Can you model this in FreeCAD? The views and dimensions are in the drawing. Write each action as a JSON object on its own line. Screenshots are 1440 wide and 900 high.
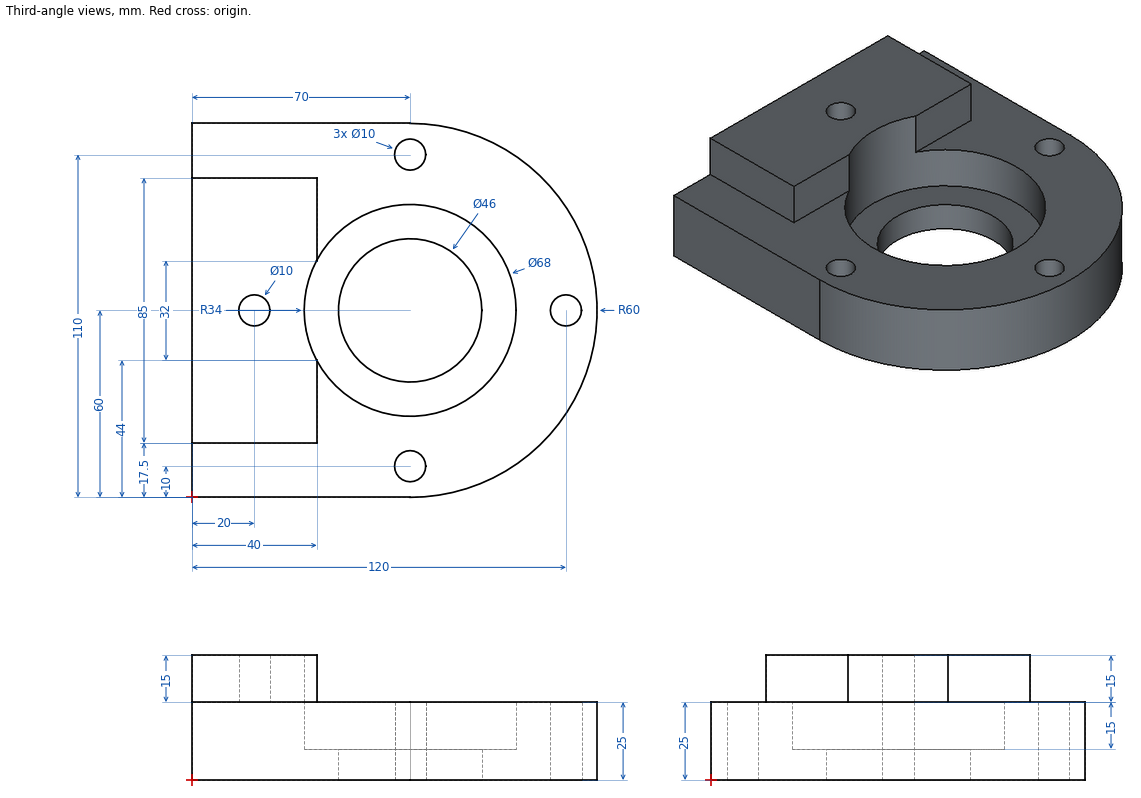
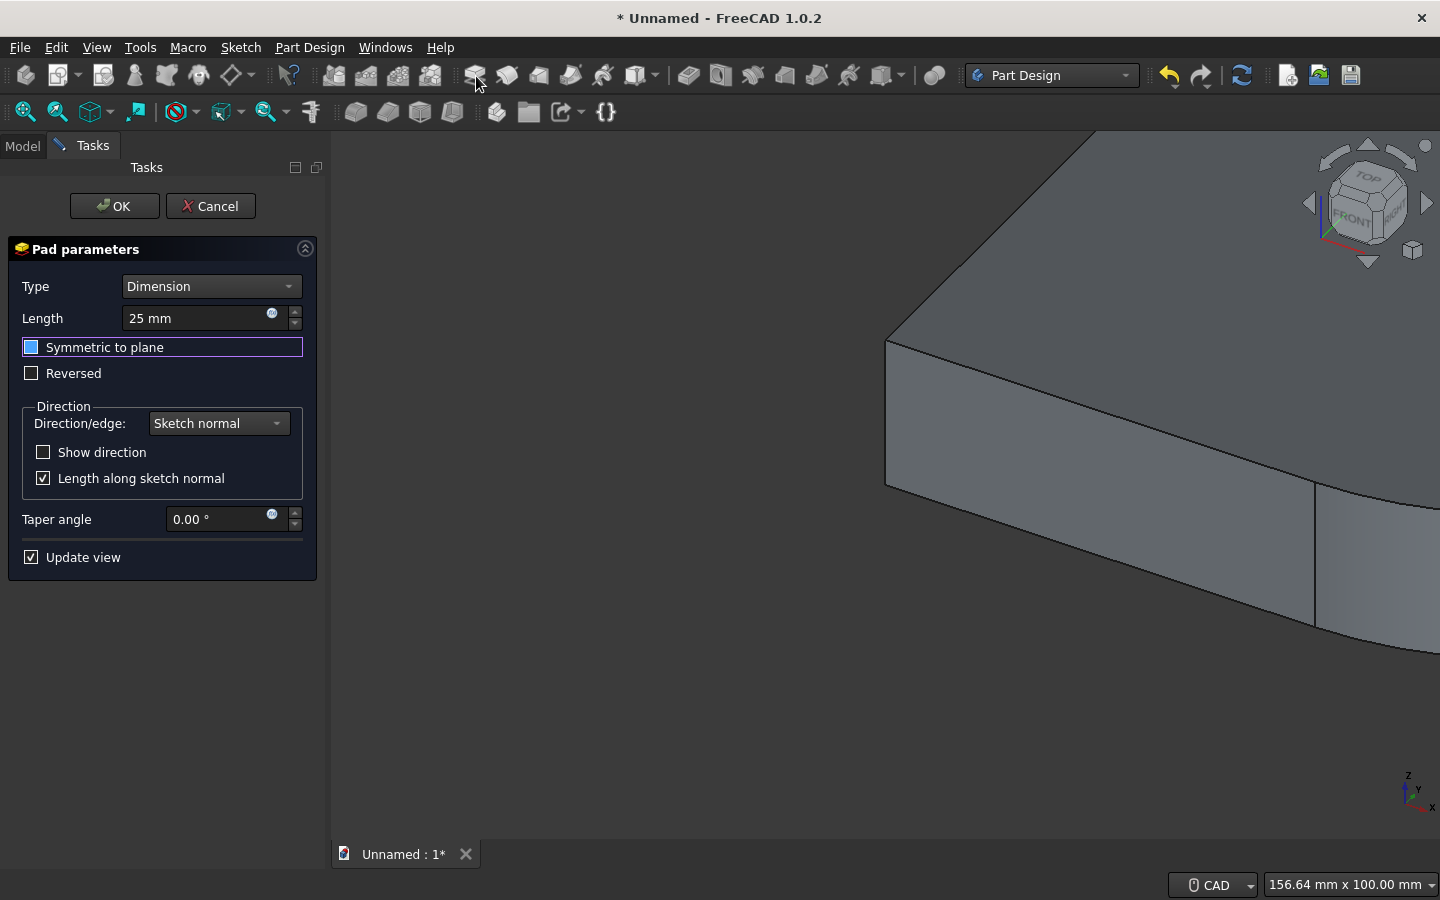
{"action": "left_click", "coordinate": [115, 206]}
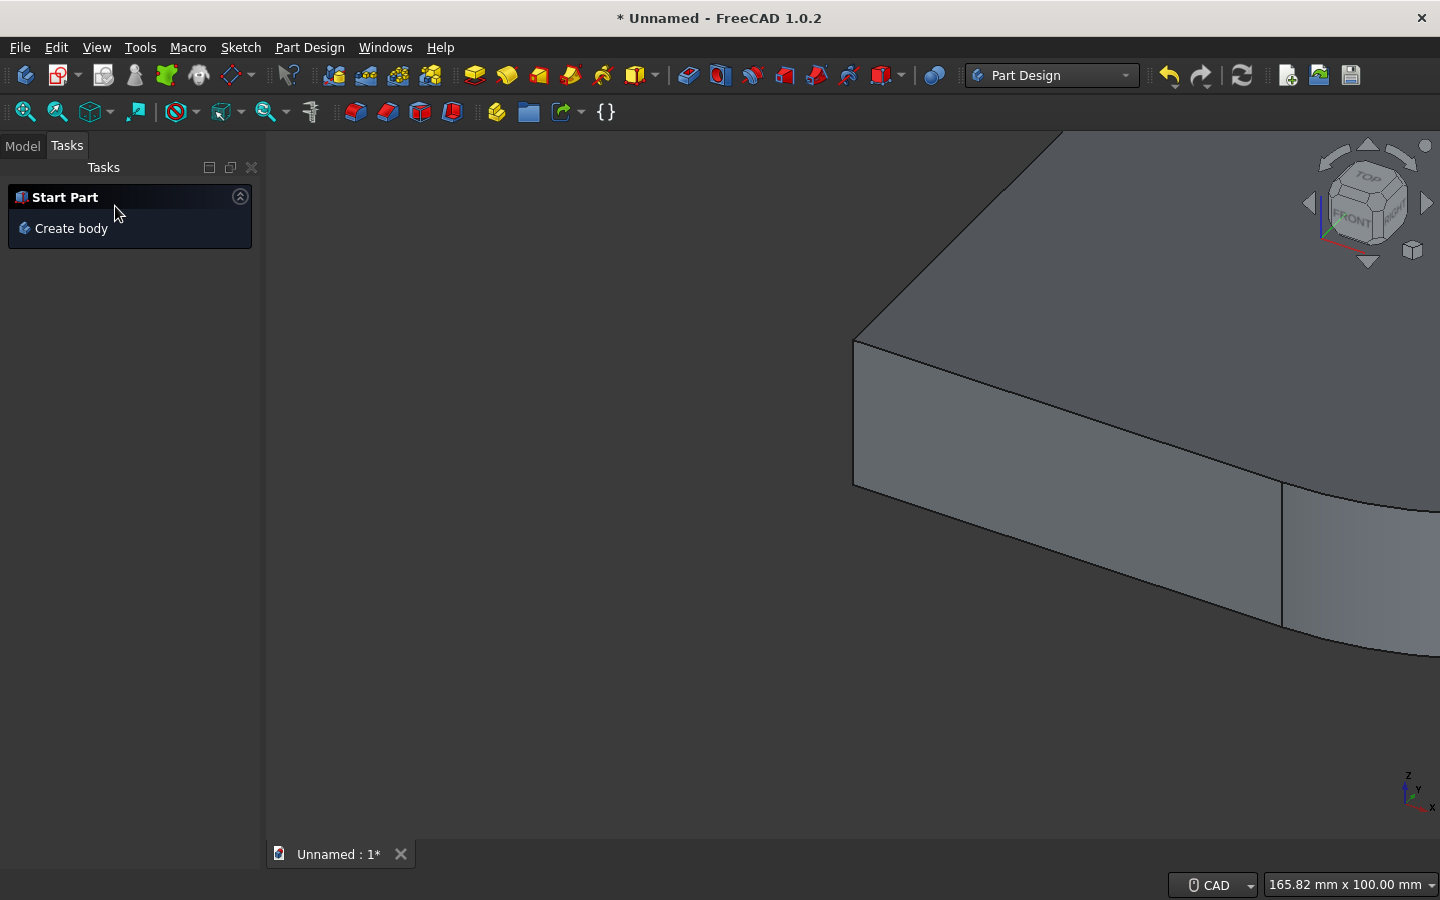
{"action": "left_click", "coordinate": [26, 112]}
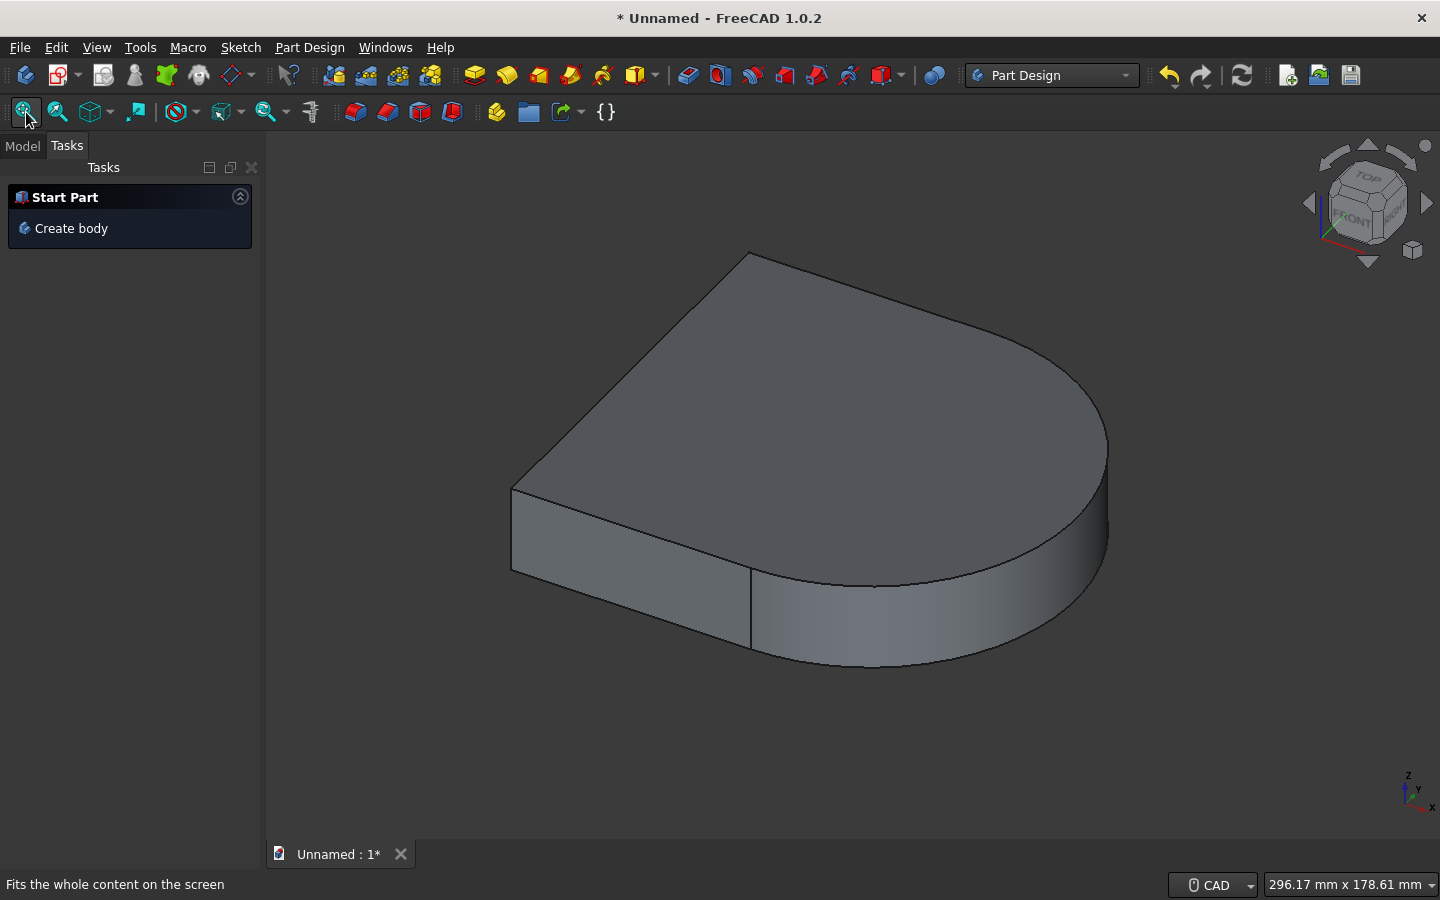
{"action": "left_click", "coordinate": [853, 443]}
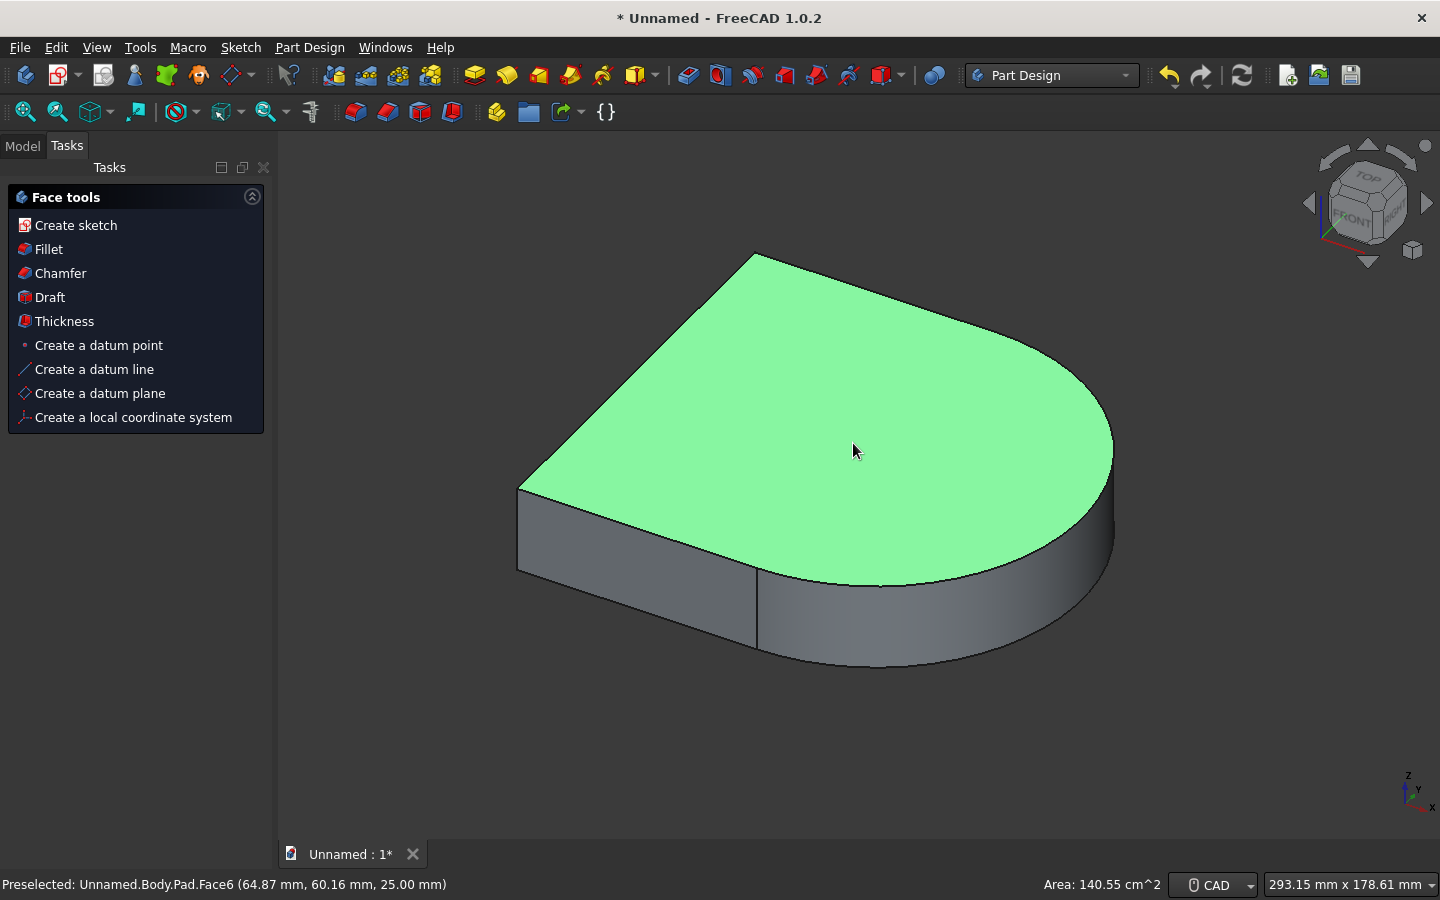
{"action": "left_click", "coordinate": [58, 76]}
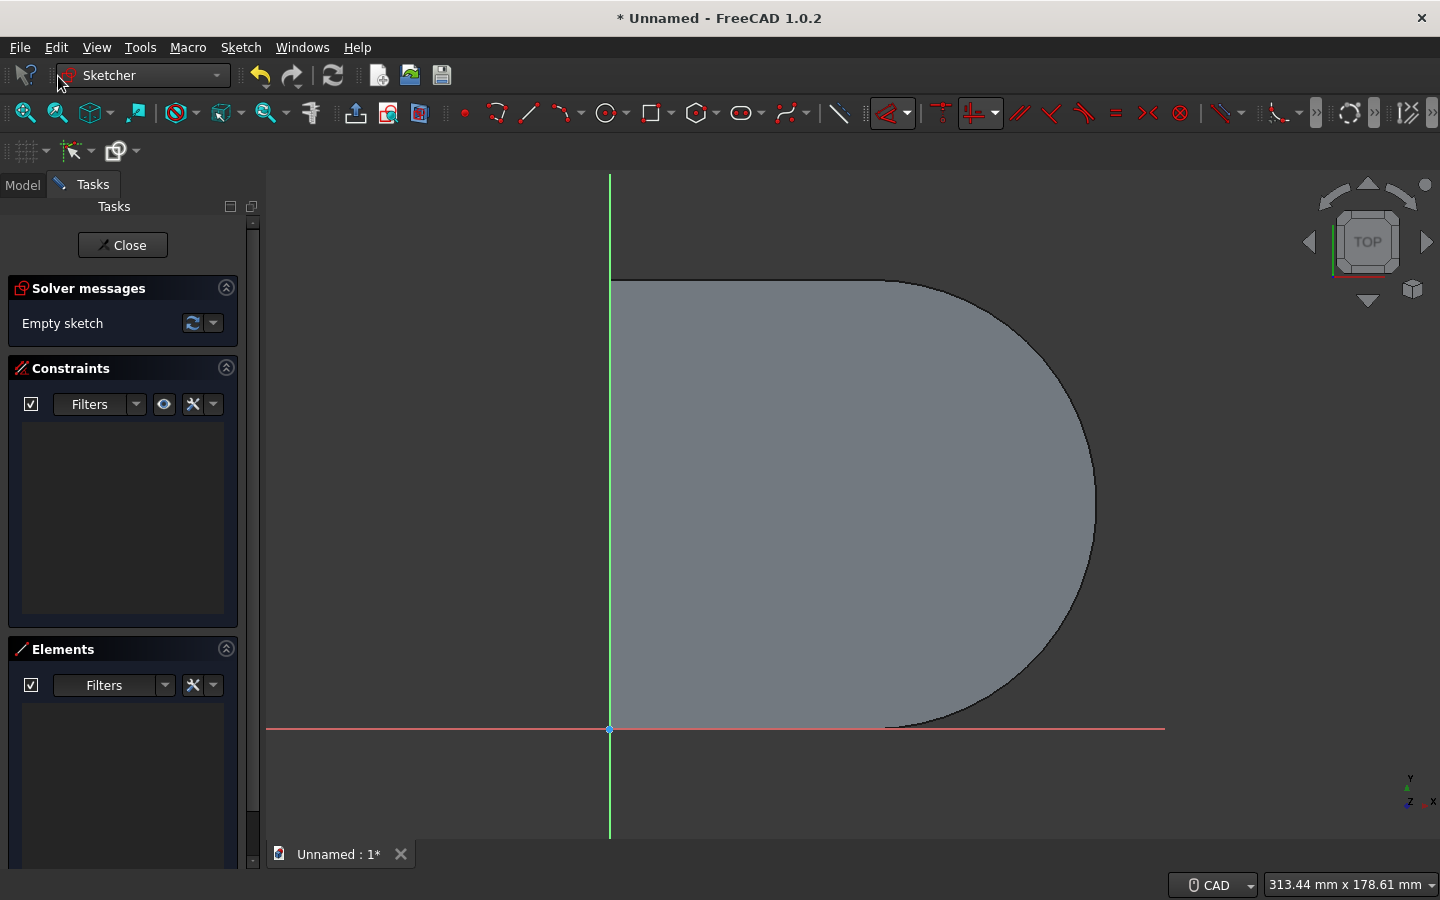
{"action": "key", "text": "g r"}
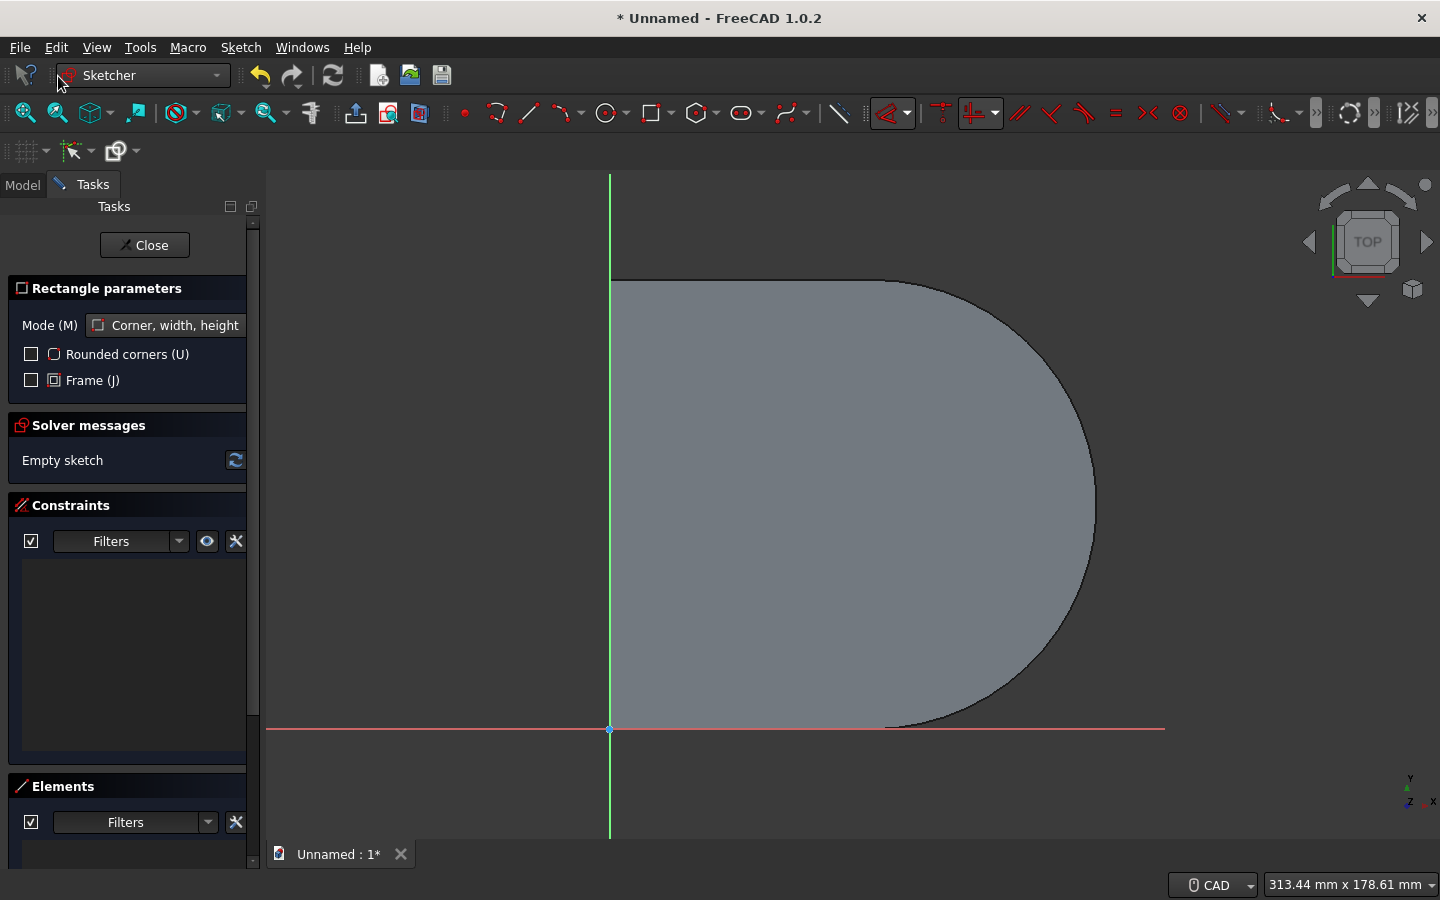
{"action": "left_click", "coordinate": [610, 345]}
{"action": "left_click", "coordinate": [760, 664]}
{"action": "key", "text": "Escape"}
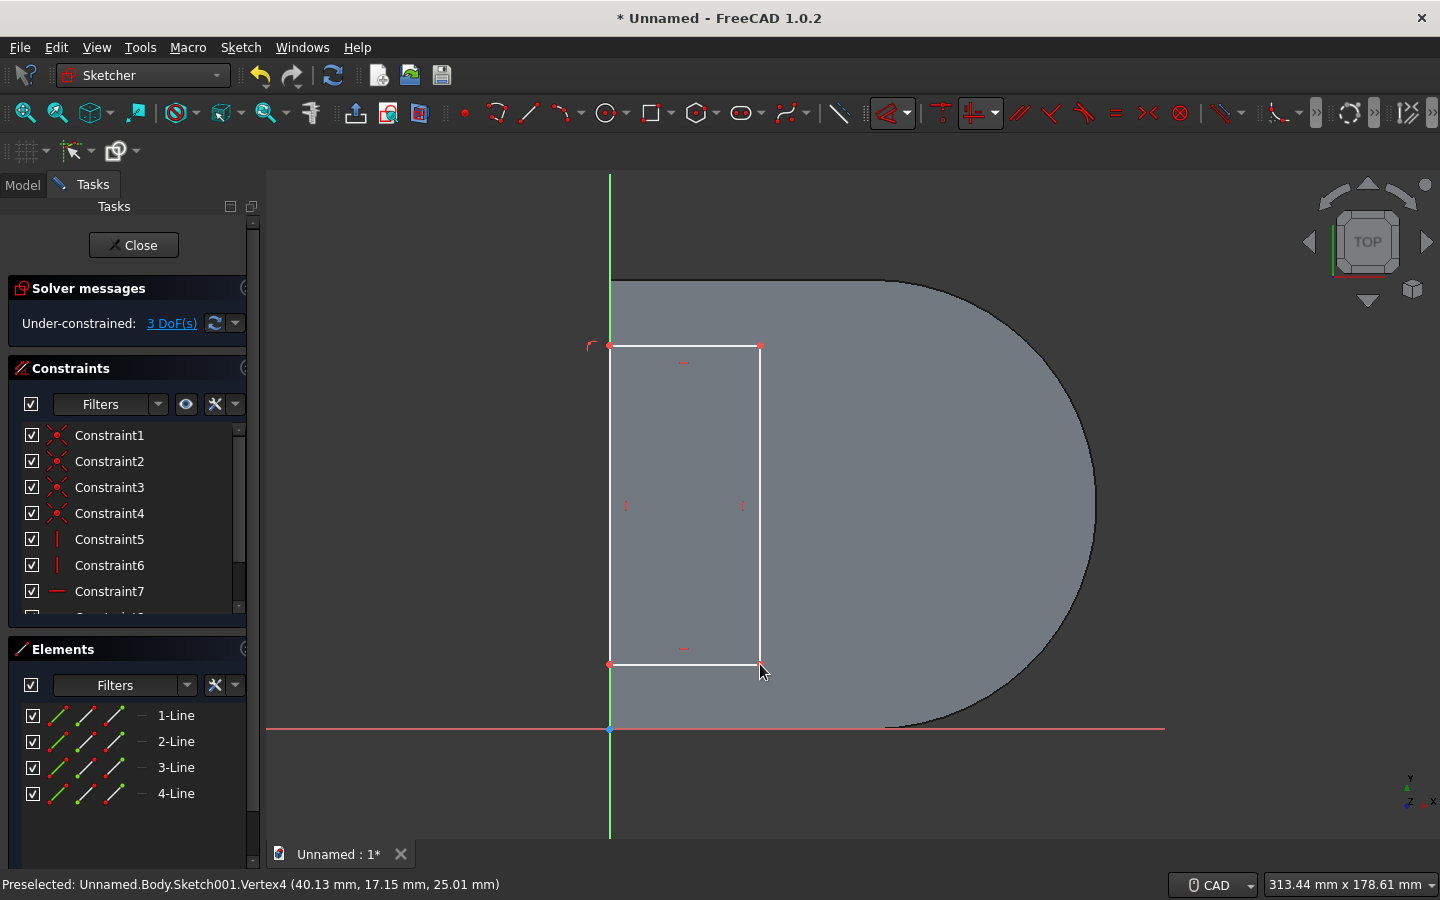
{"action": "left_click", "coordinate": [610, 442]}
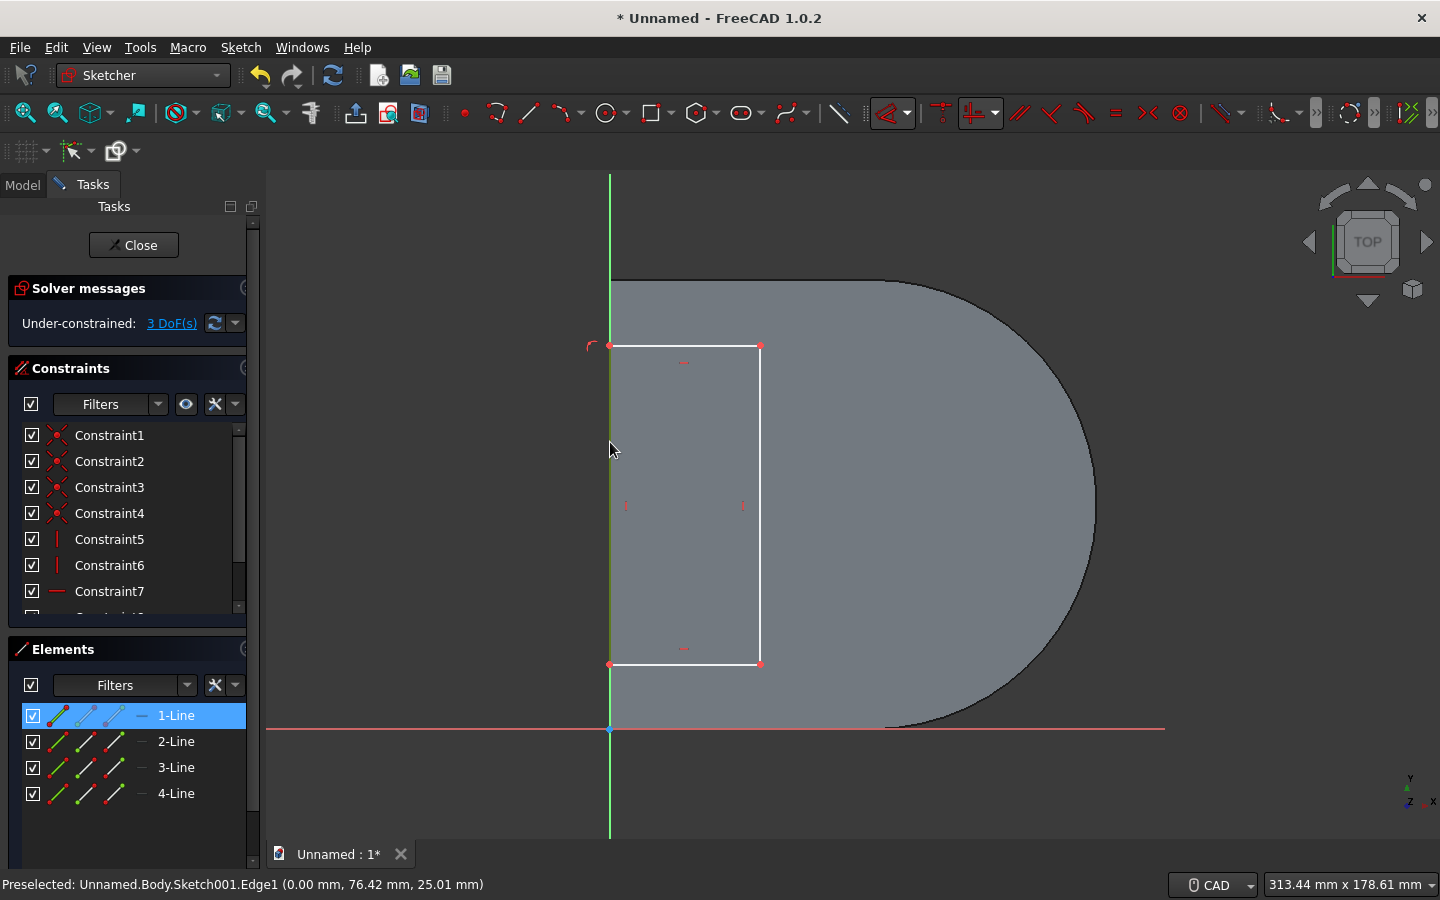
{"action": "key", "text": "i"}